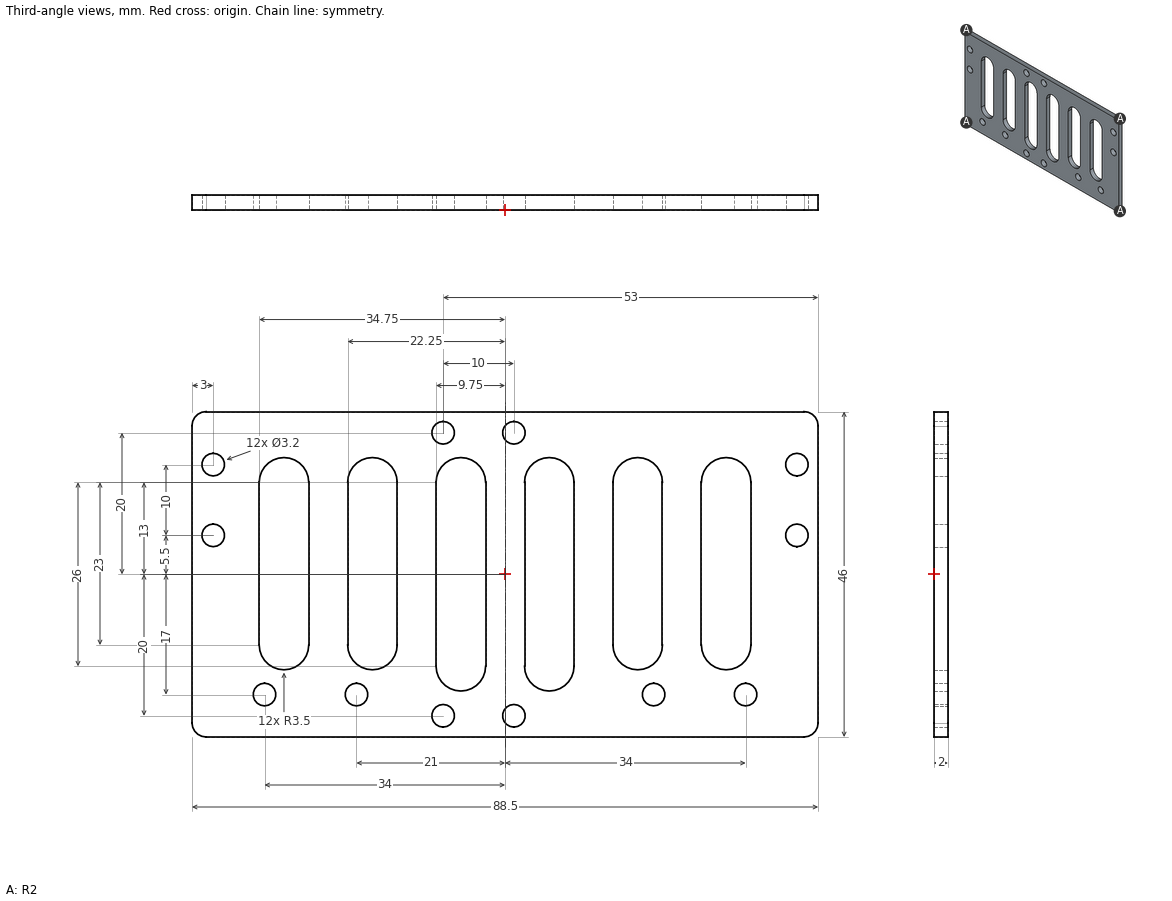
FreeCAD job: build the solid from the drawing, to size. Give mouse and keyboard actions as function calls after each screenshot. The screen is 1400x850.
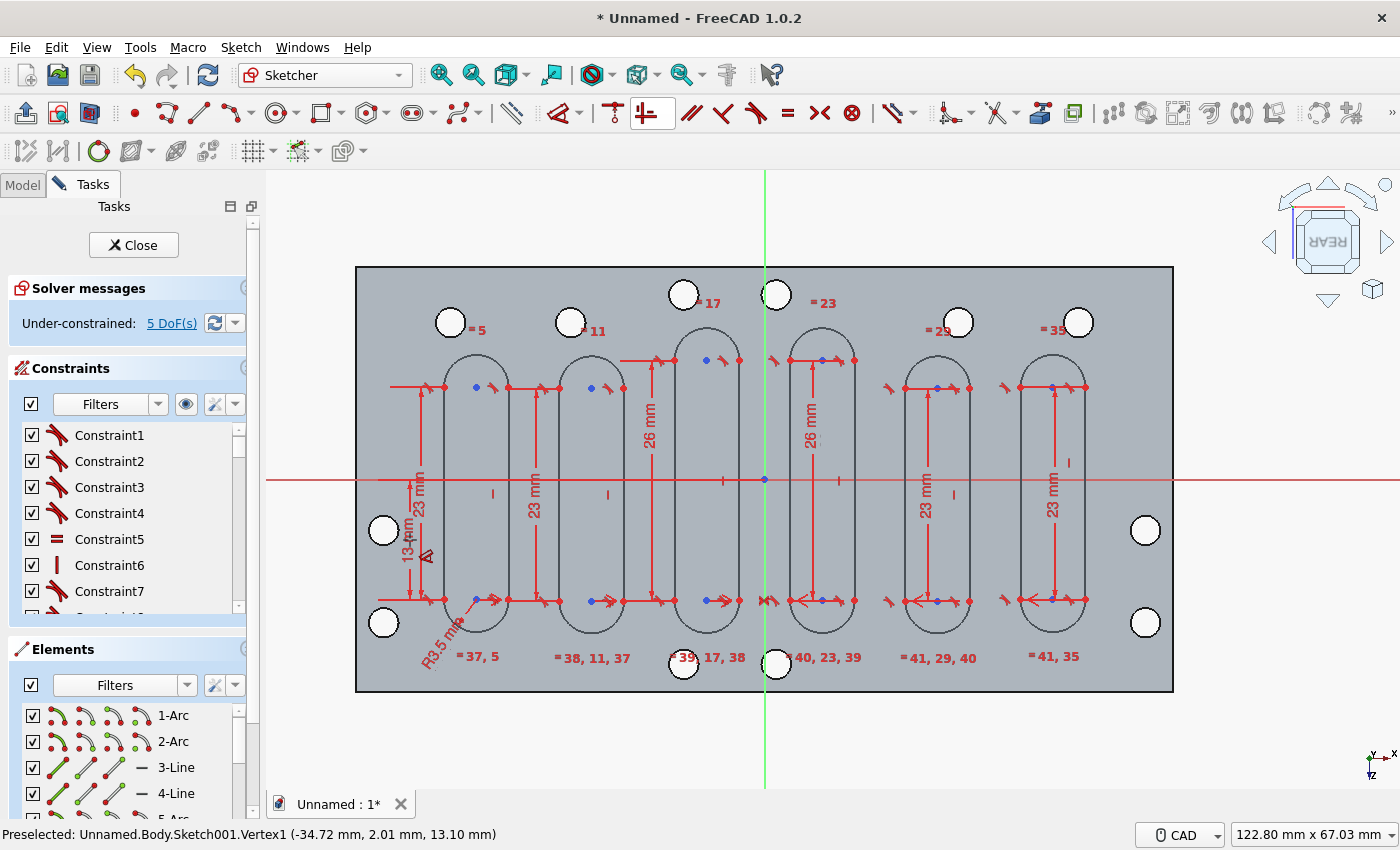
click(559, 601)
click(525, 540)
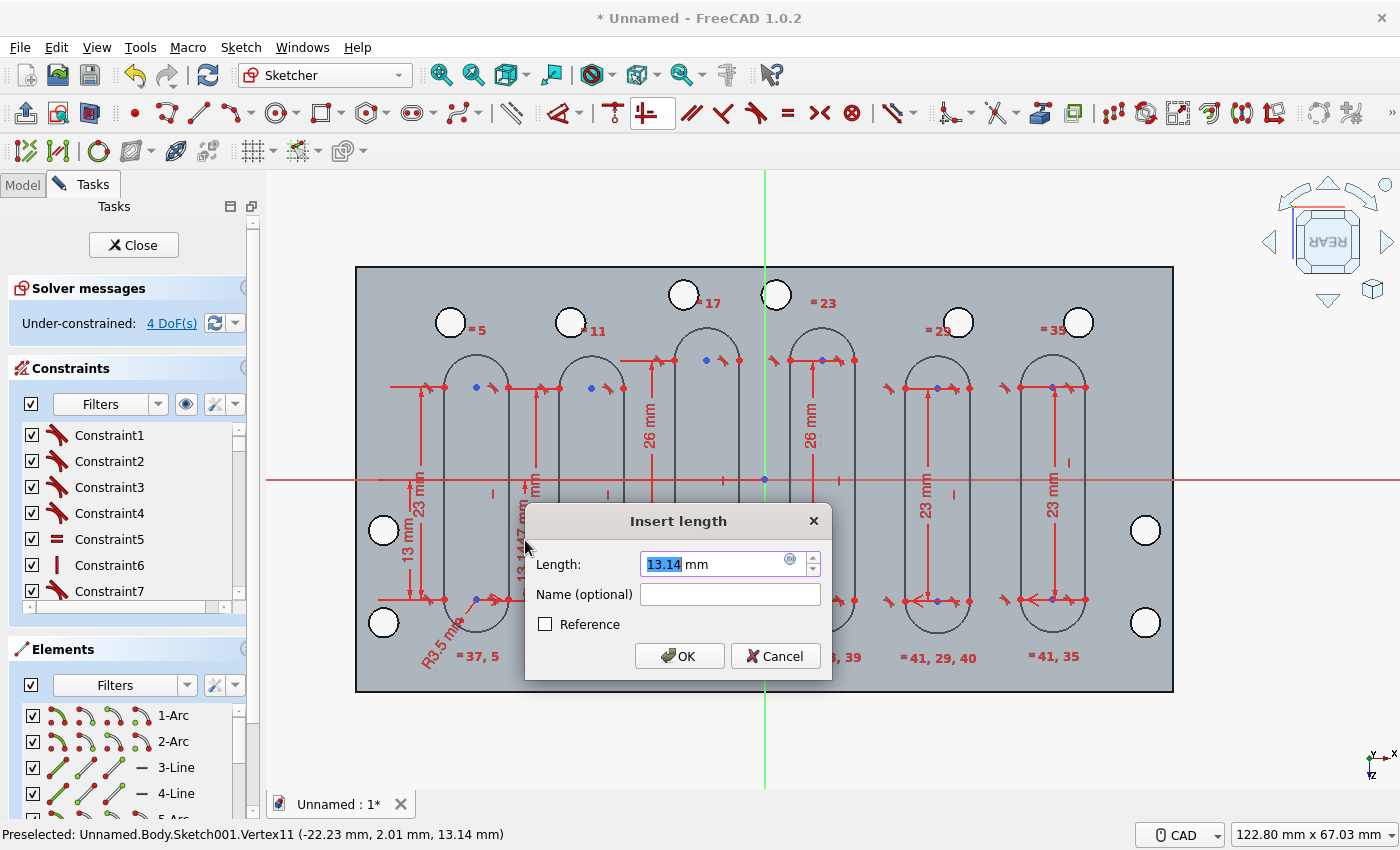
text(13)
key(Return)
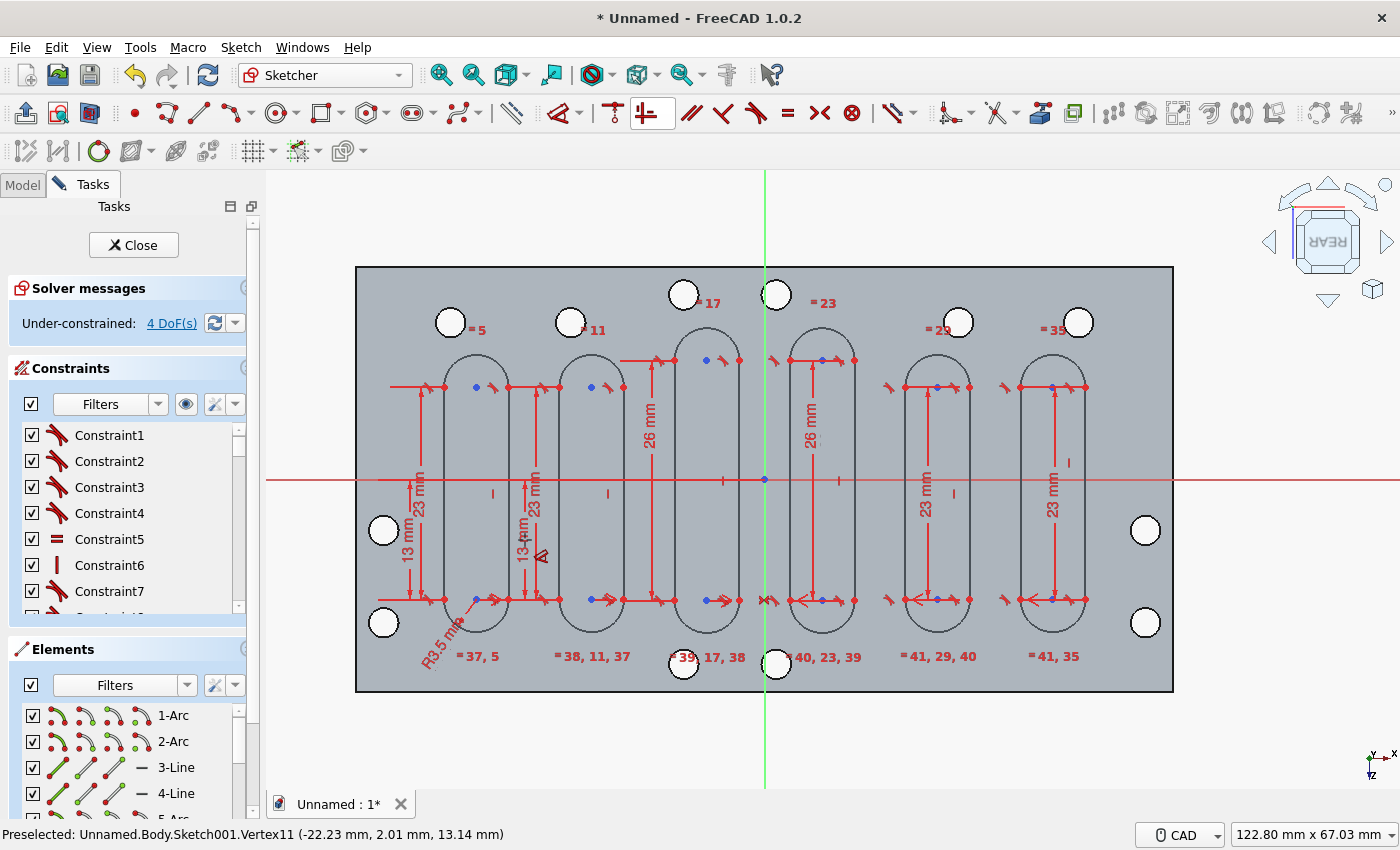
click(675, 601)
click(641, 540)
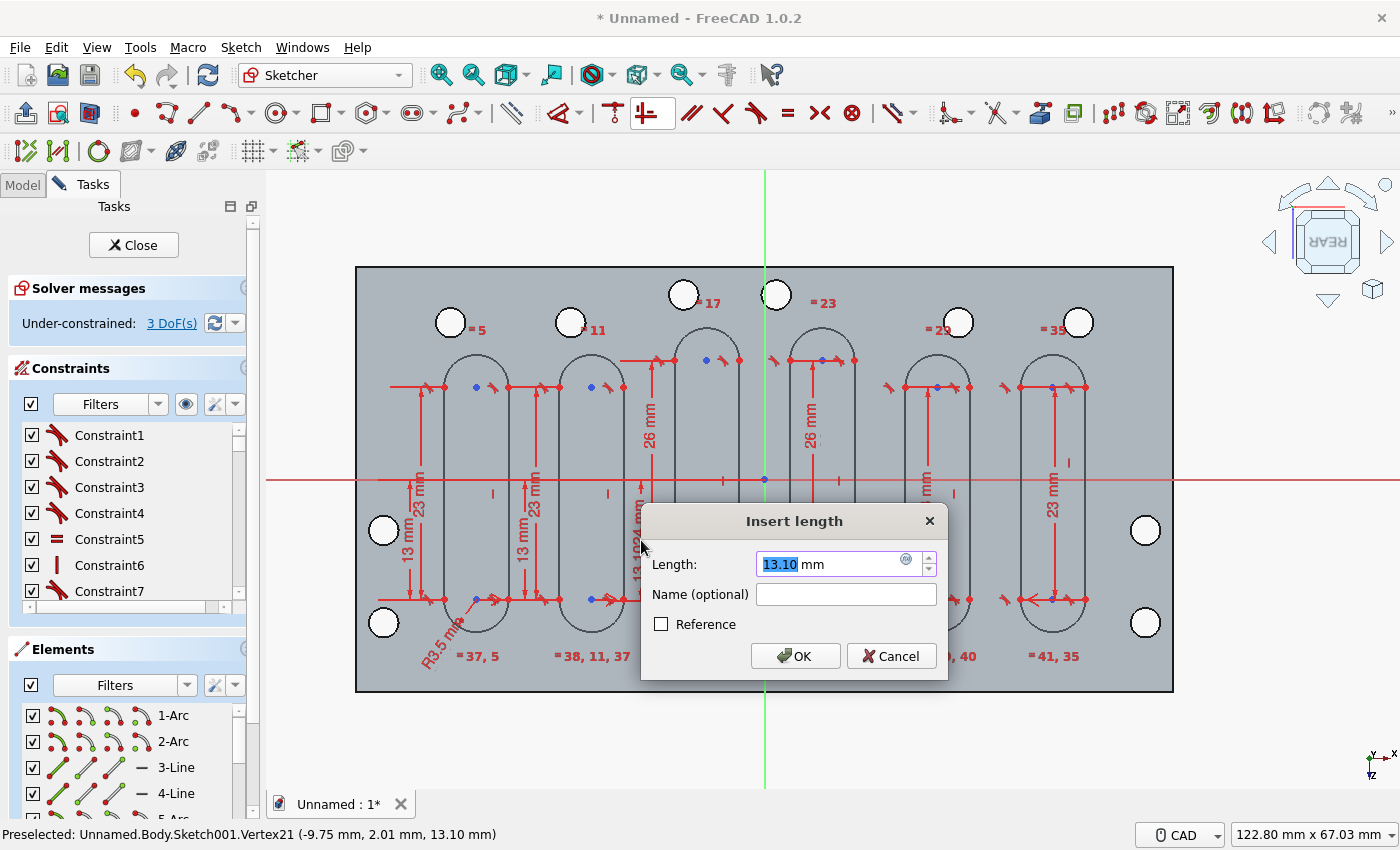
text(13)
key(Return)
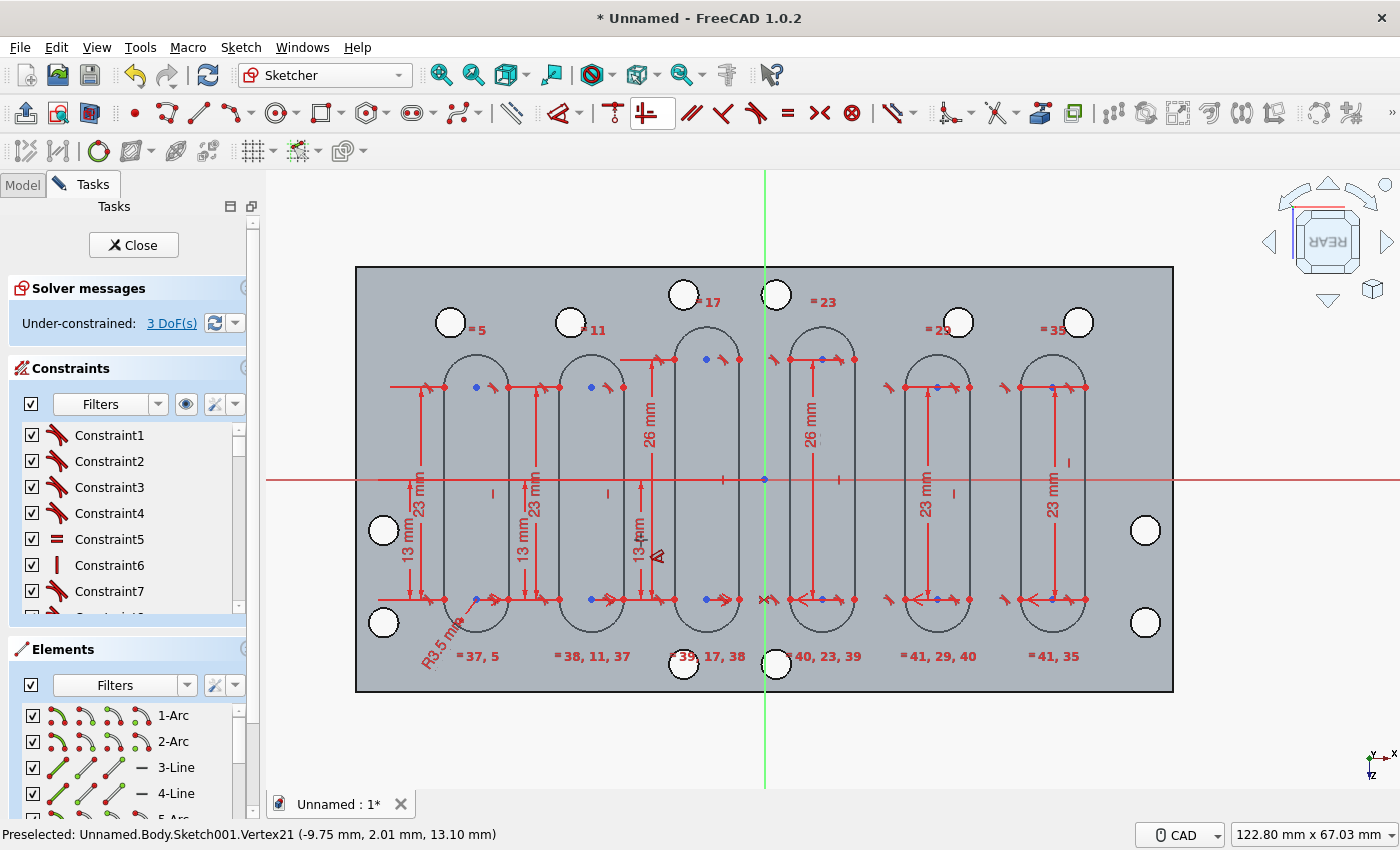
click(675, 600)
click(740, 634)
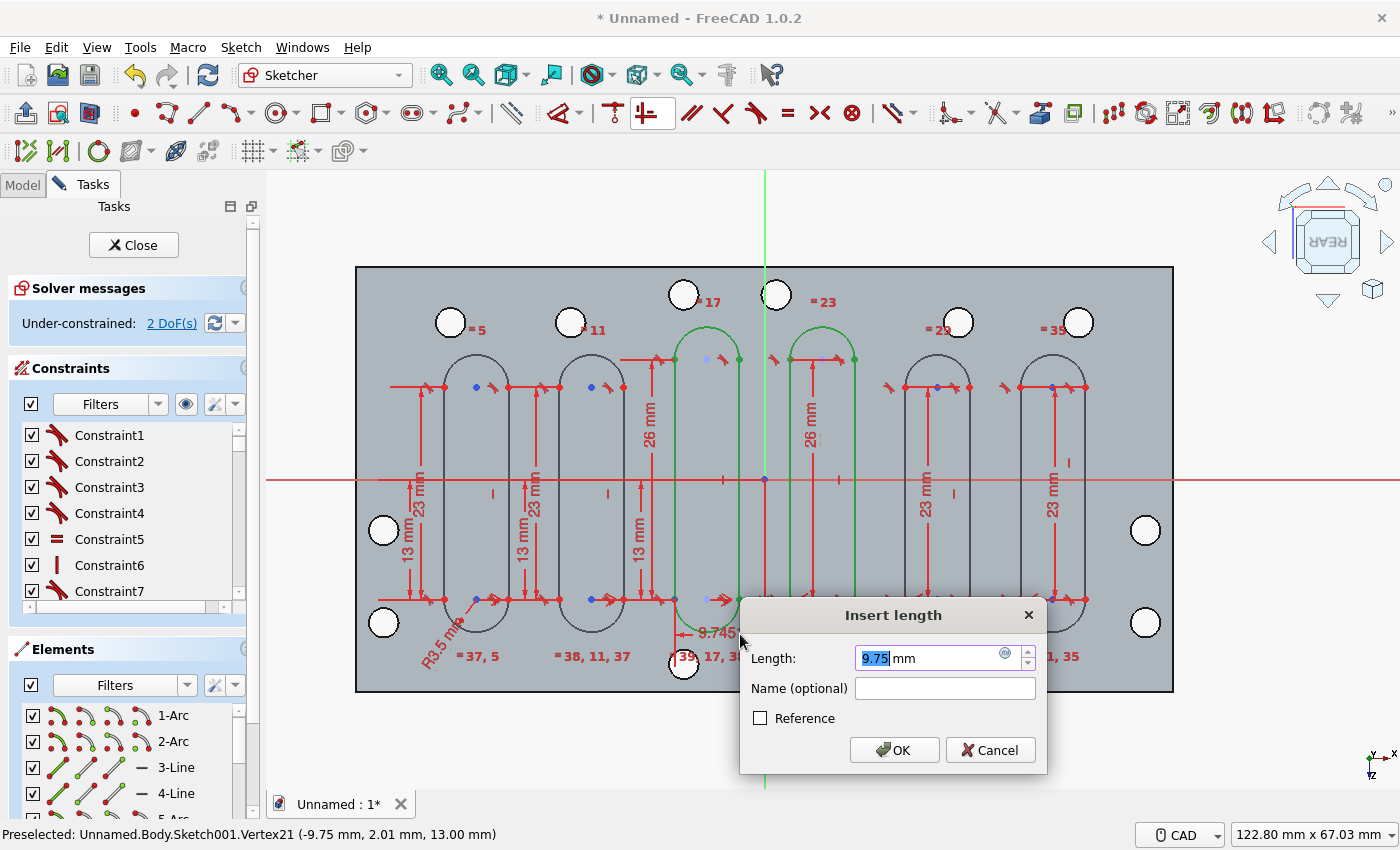
text(9.75)
key(Return)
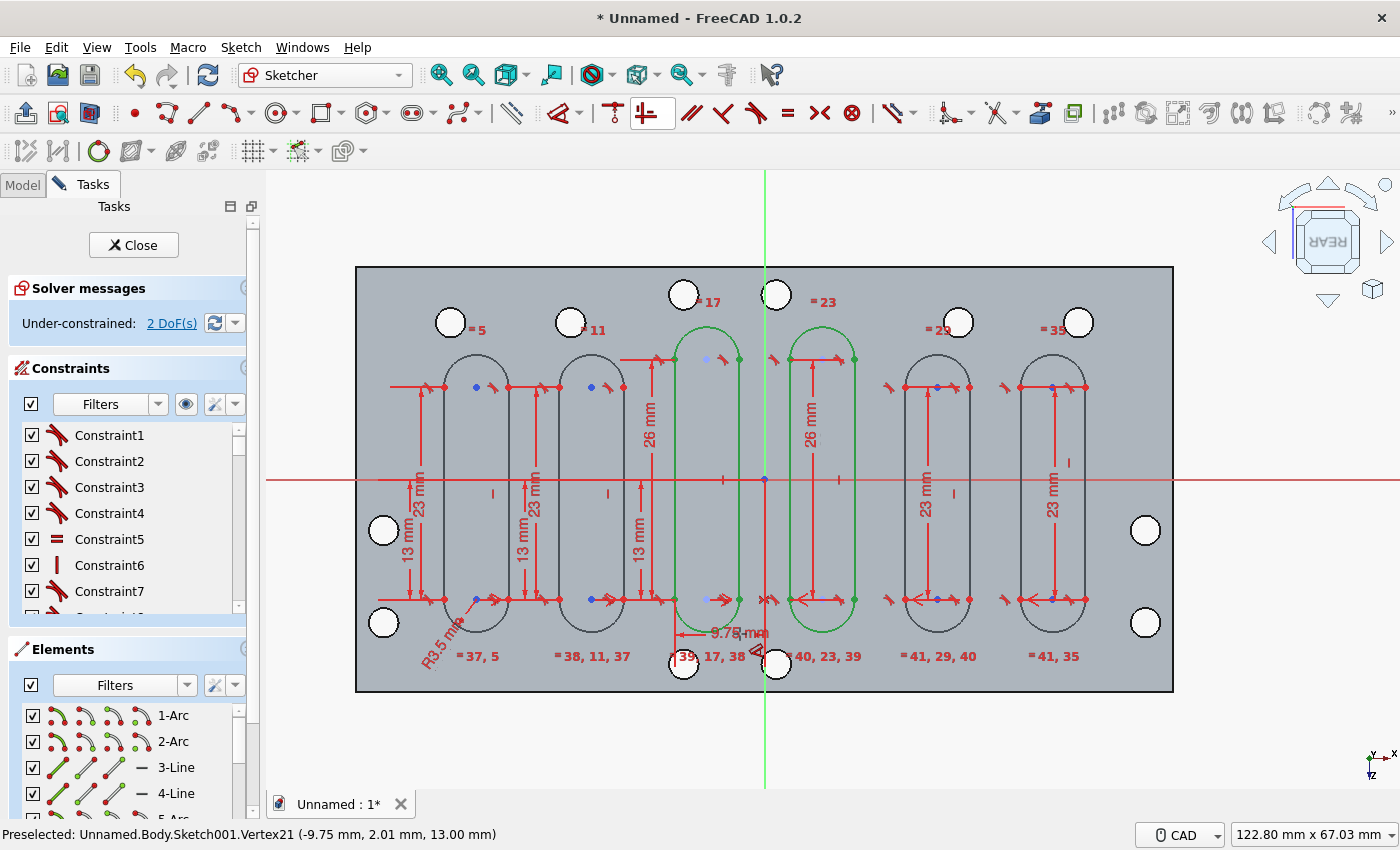
click(444, 600)
click(531, 634)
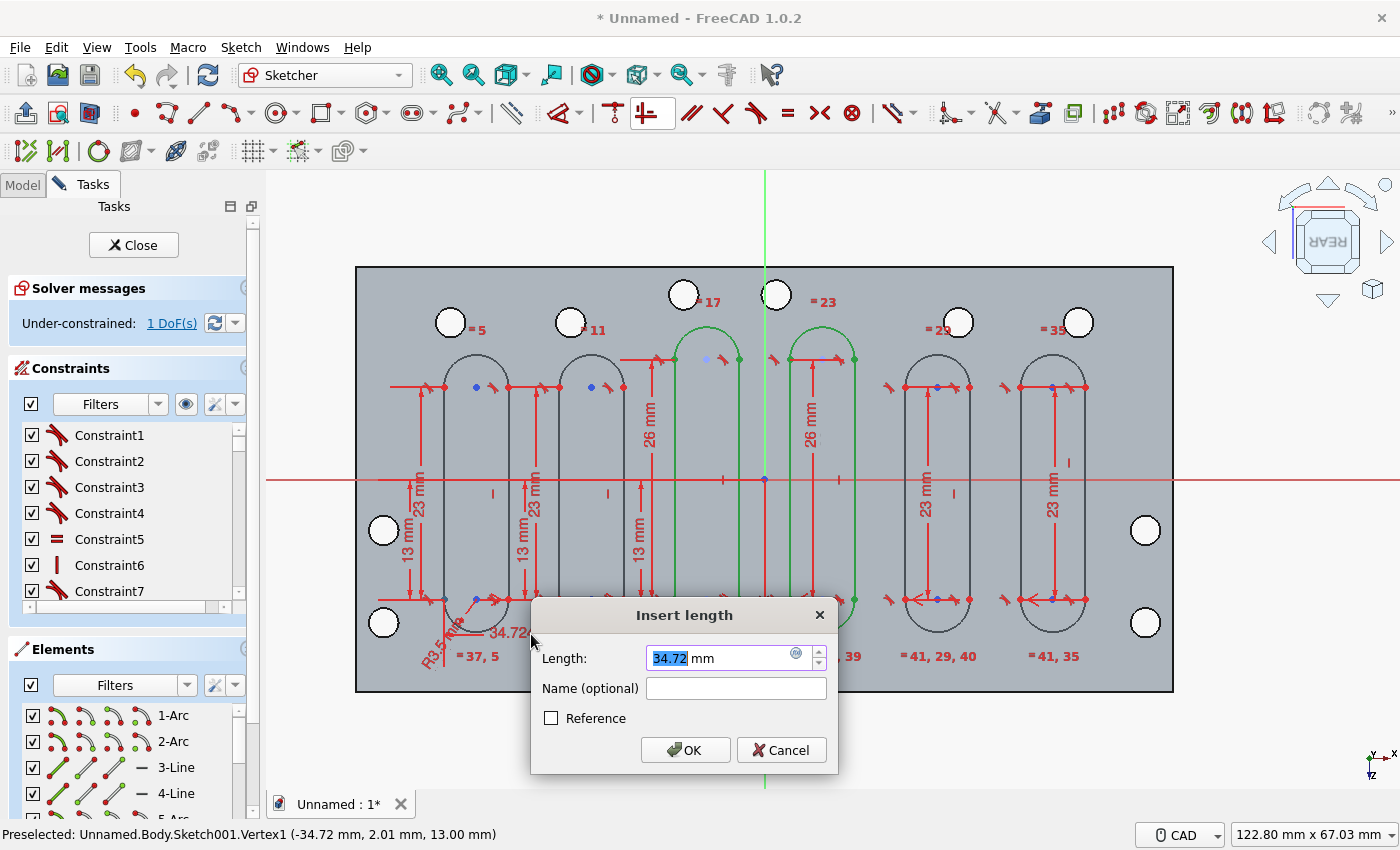
text(34.75)
key(Return)